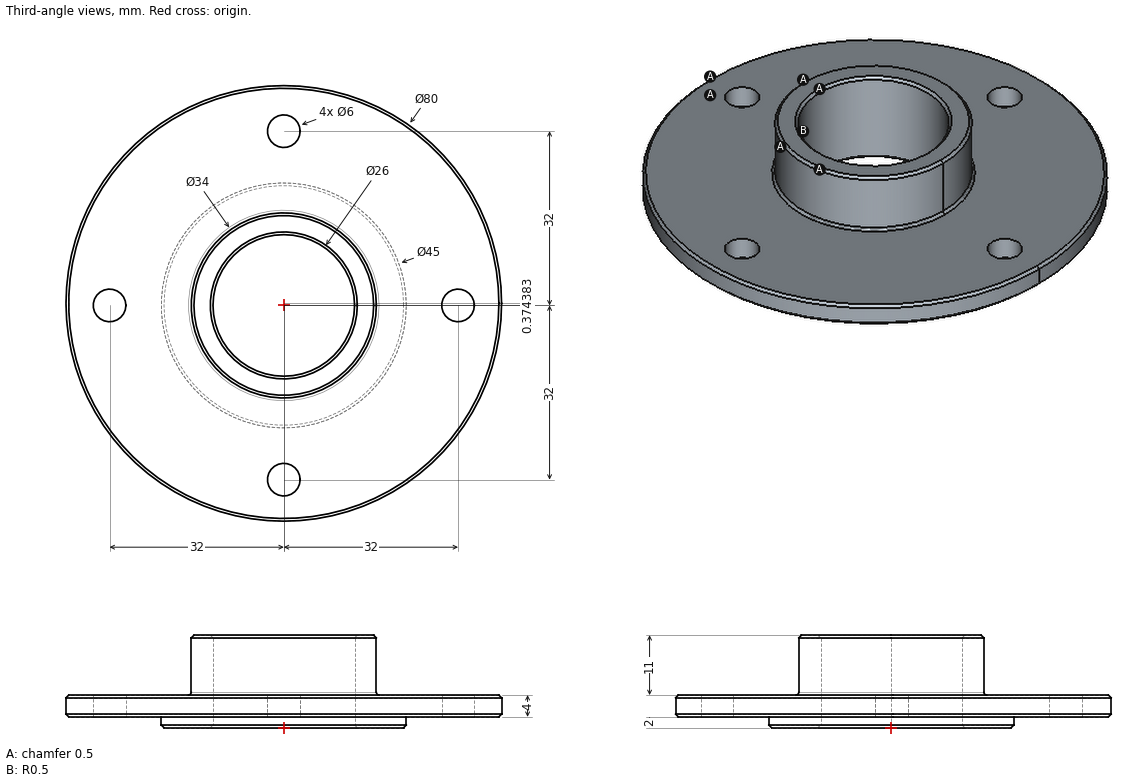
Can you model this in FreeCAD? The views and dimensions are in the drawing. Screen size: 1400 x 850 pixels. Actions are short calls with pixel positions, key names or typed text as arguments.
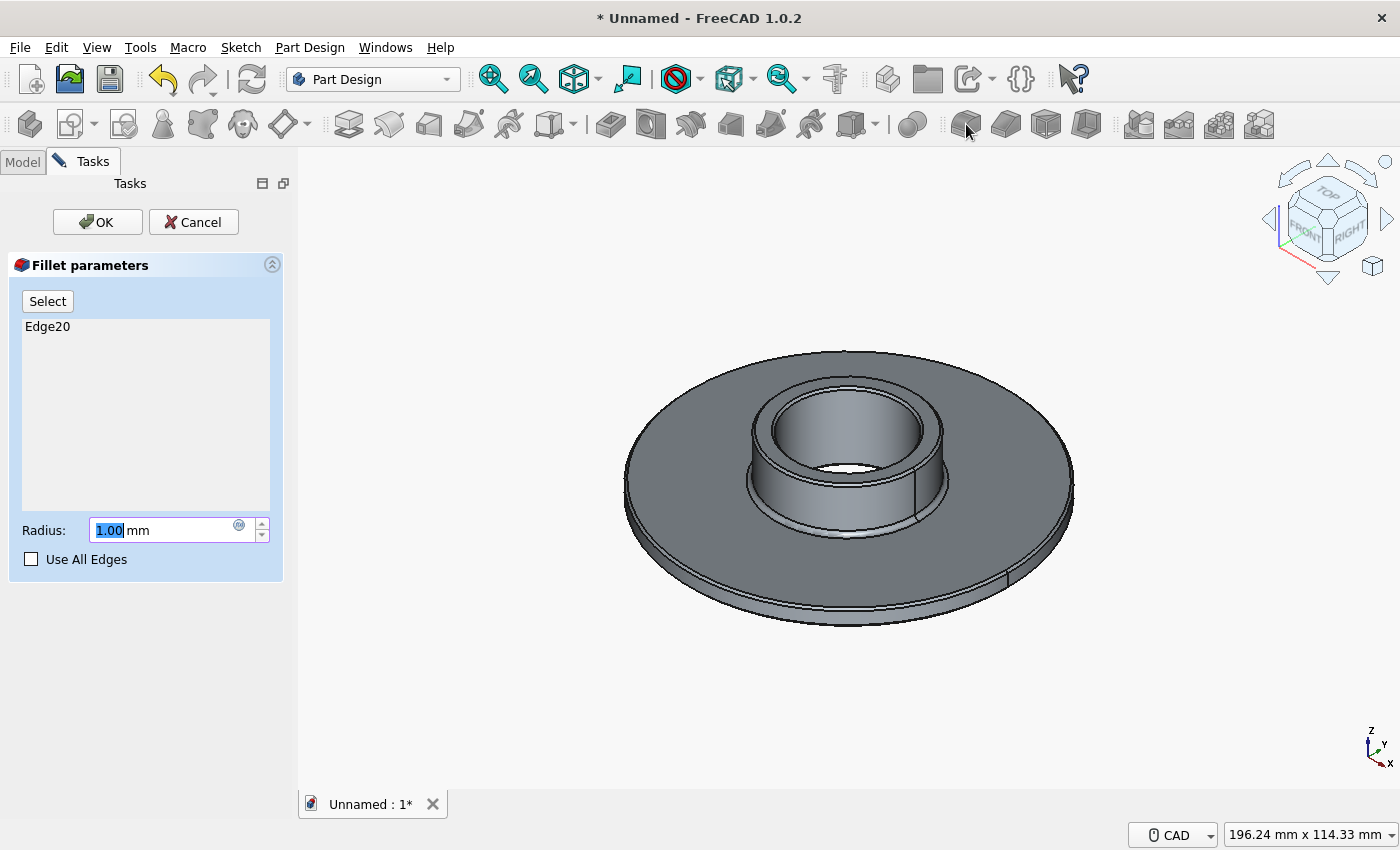
text(0.5)
key(Tab)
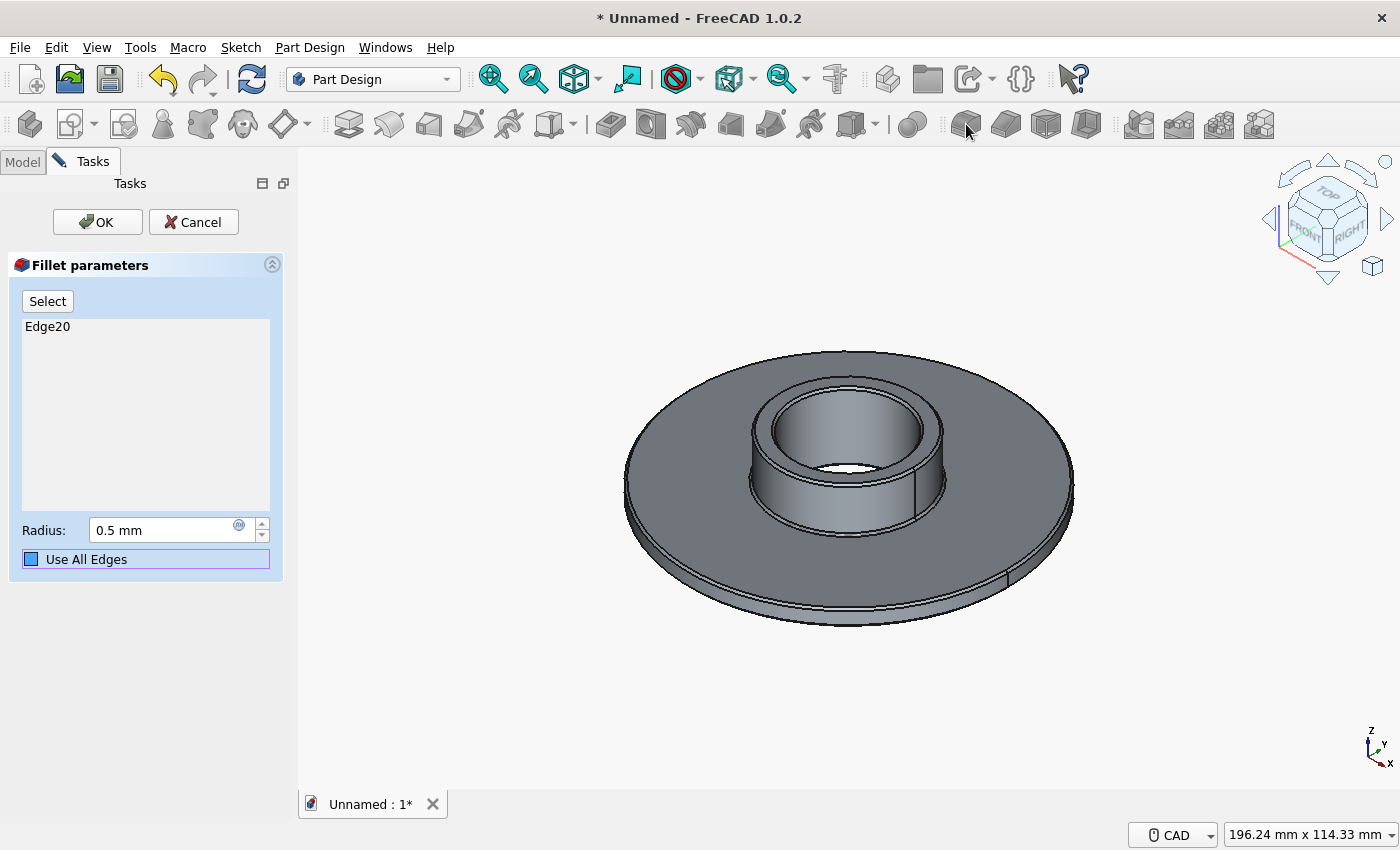
click(98, 222)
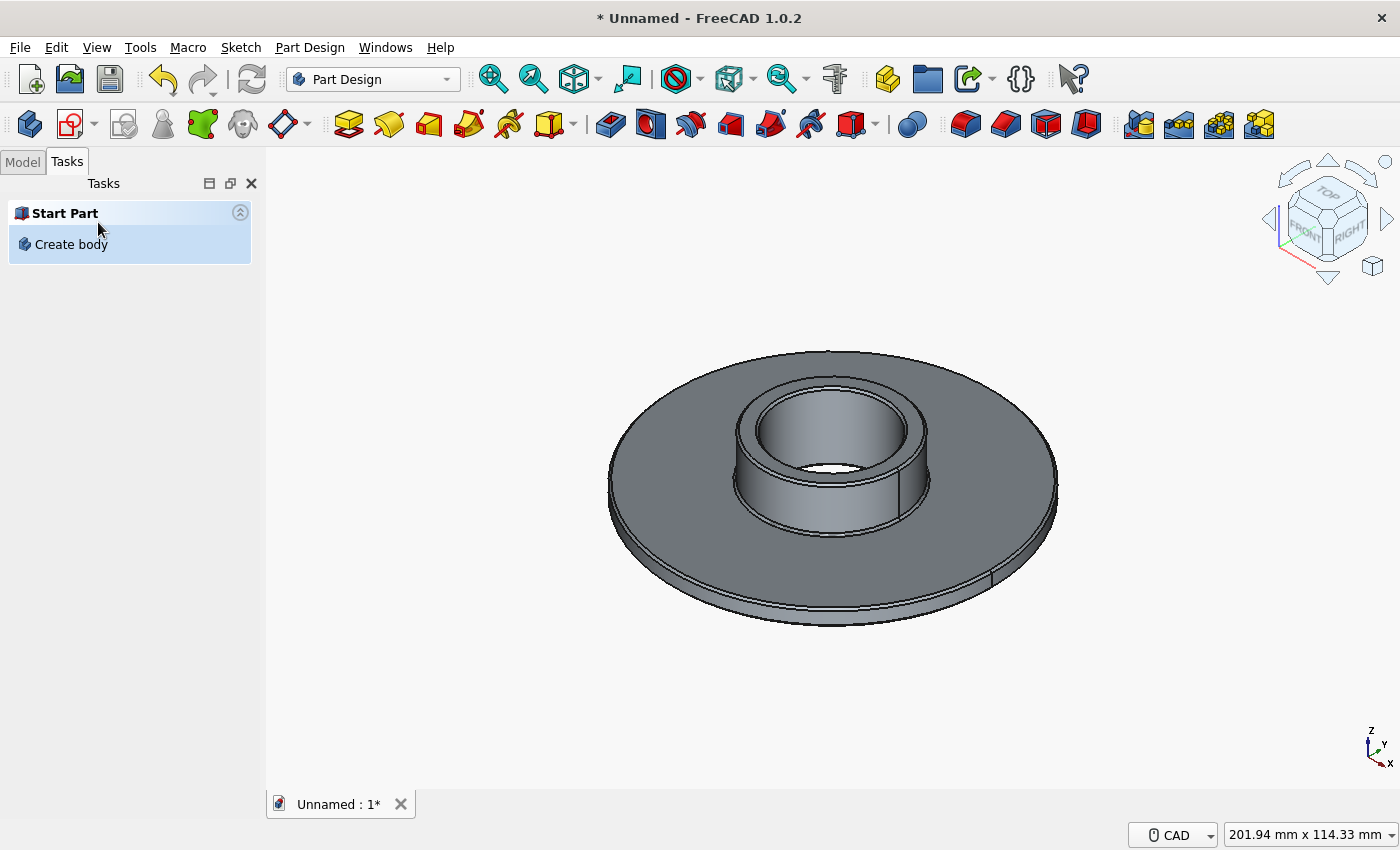
click(967, 453)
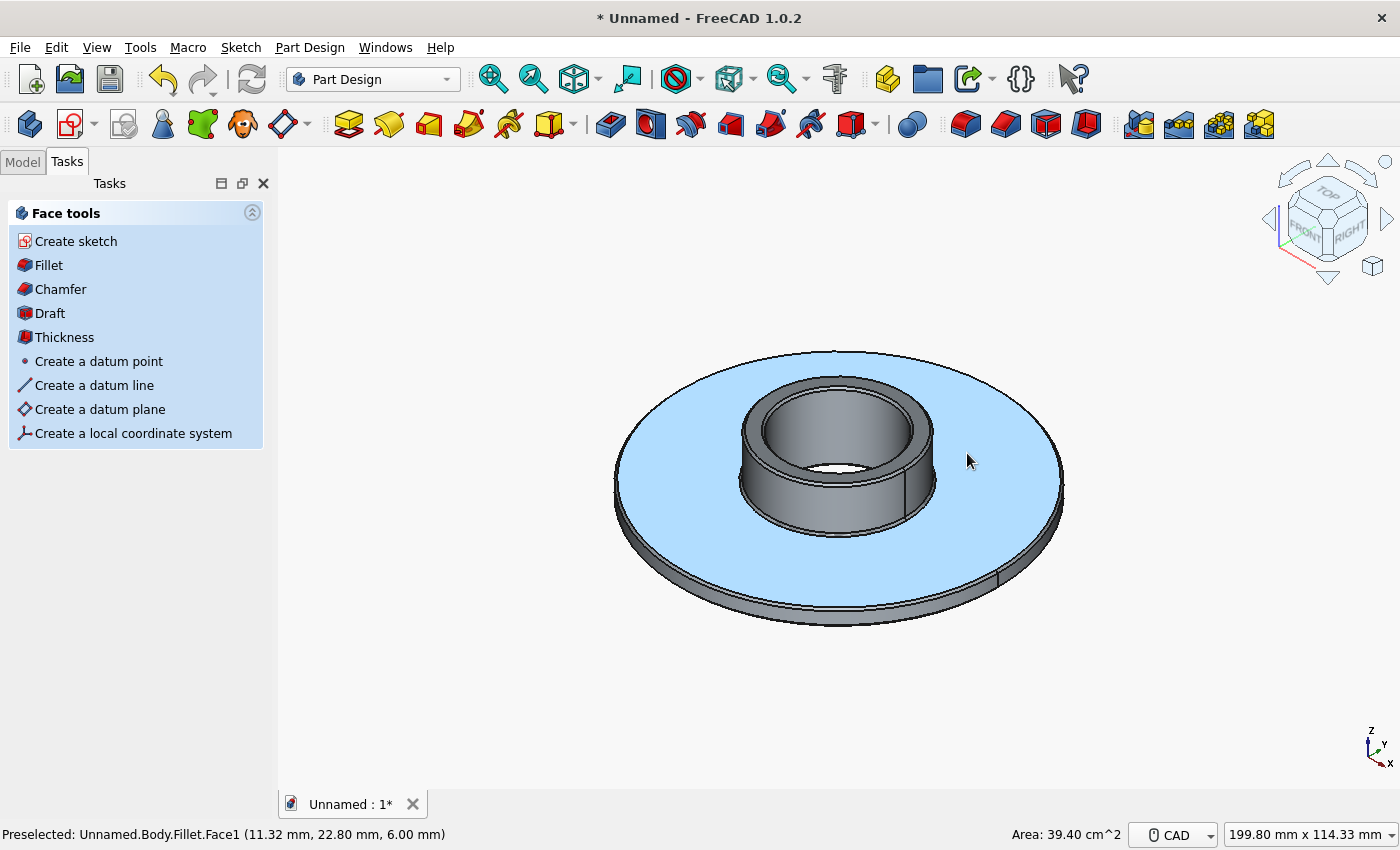
click(70, 124)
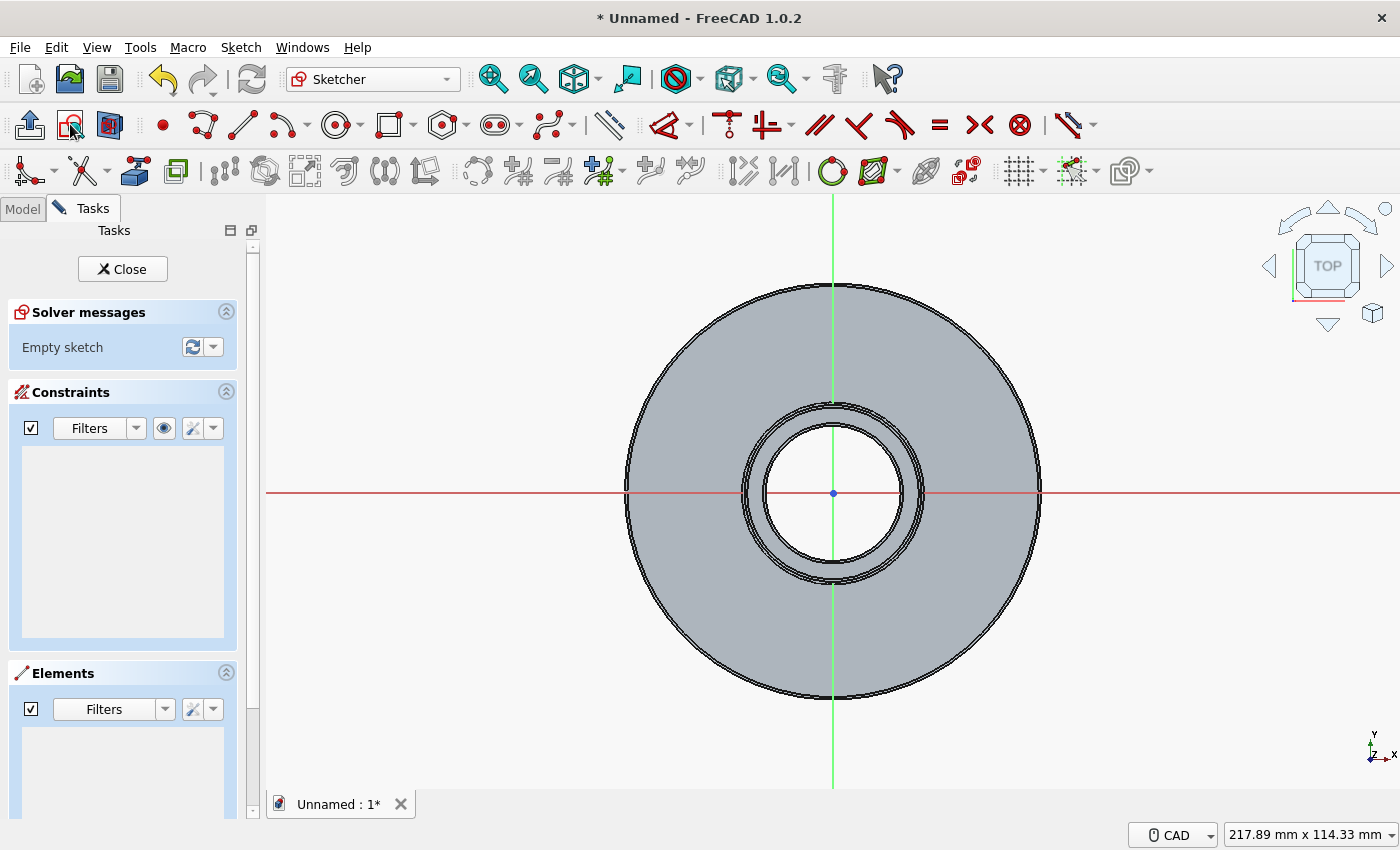
click(110, 126)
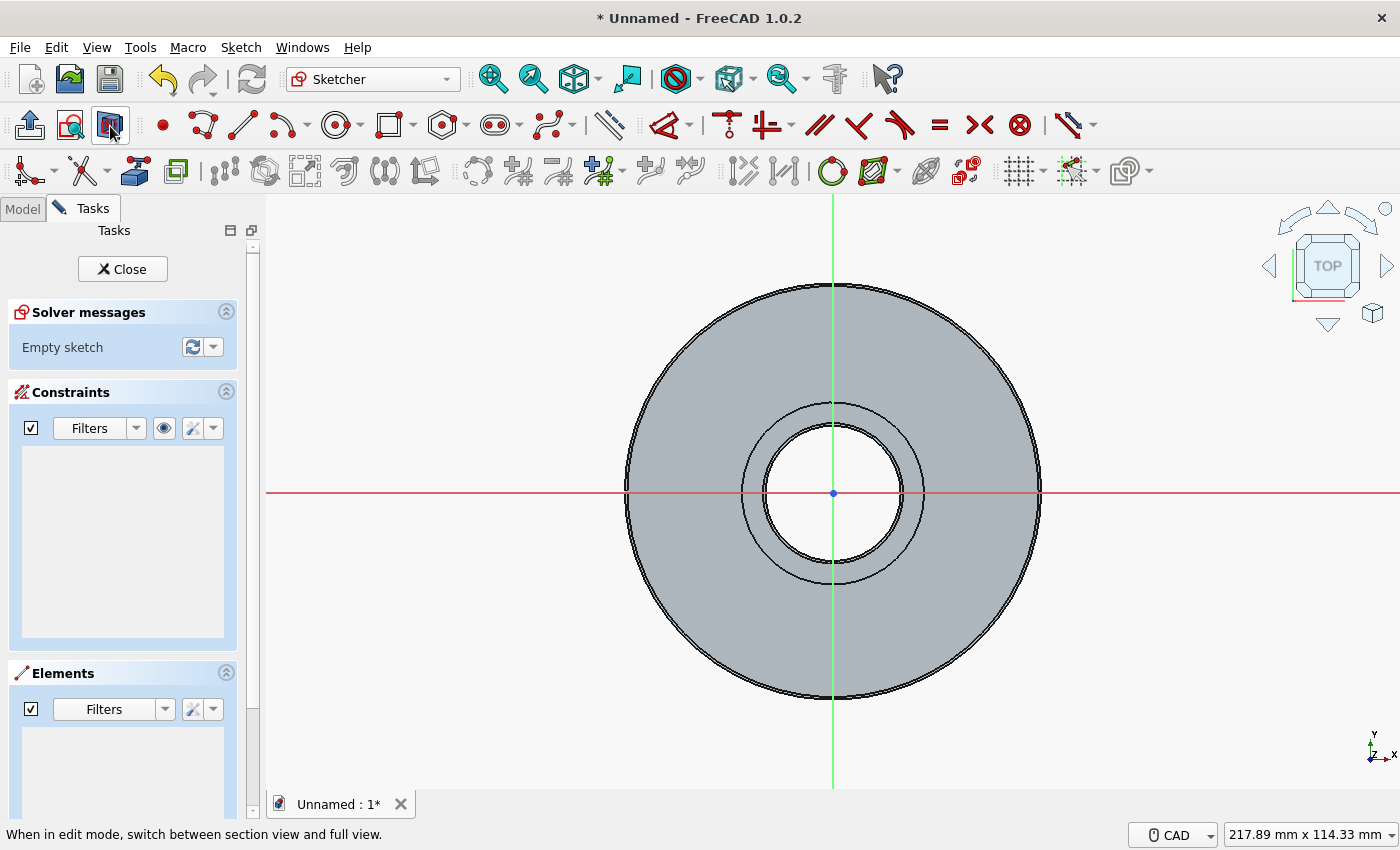
click(336, 126)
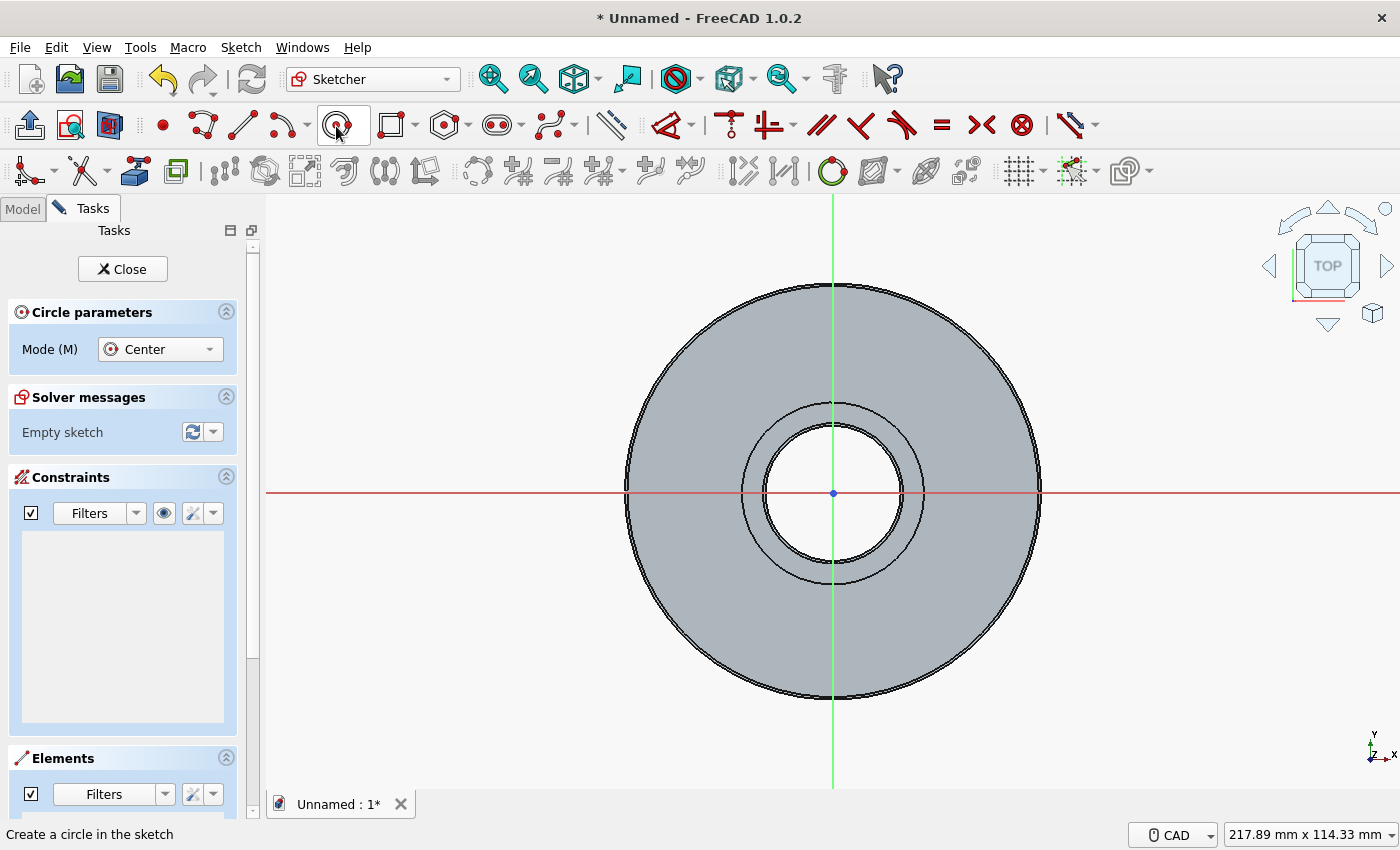
scroll(833, 327, up, 2)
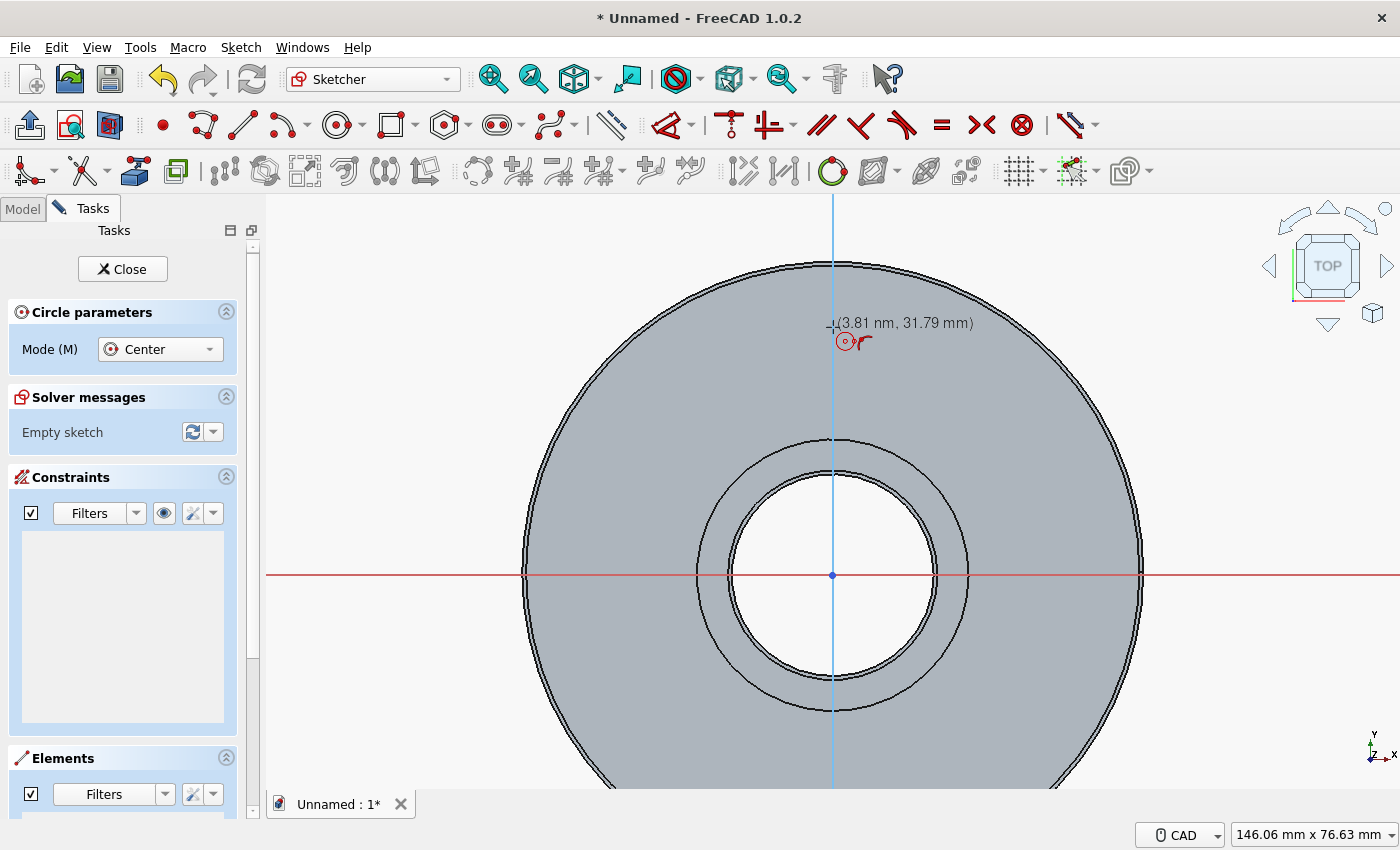
click(833, 327)
move(849, 310)